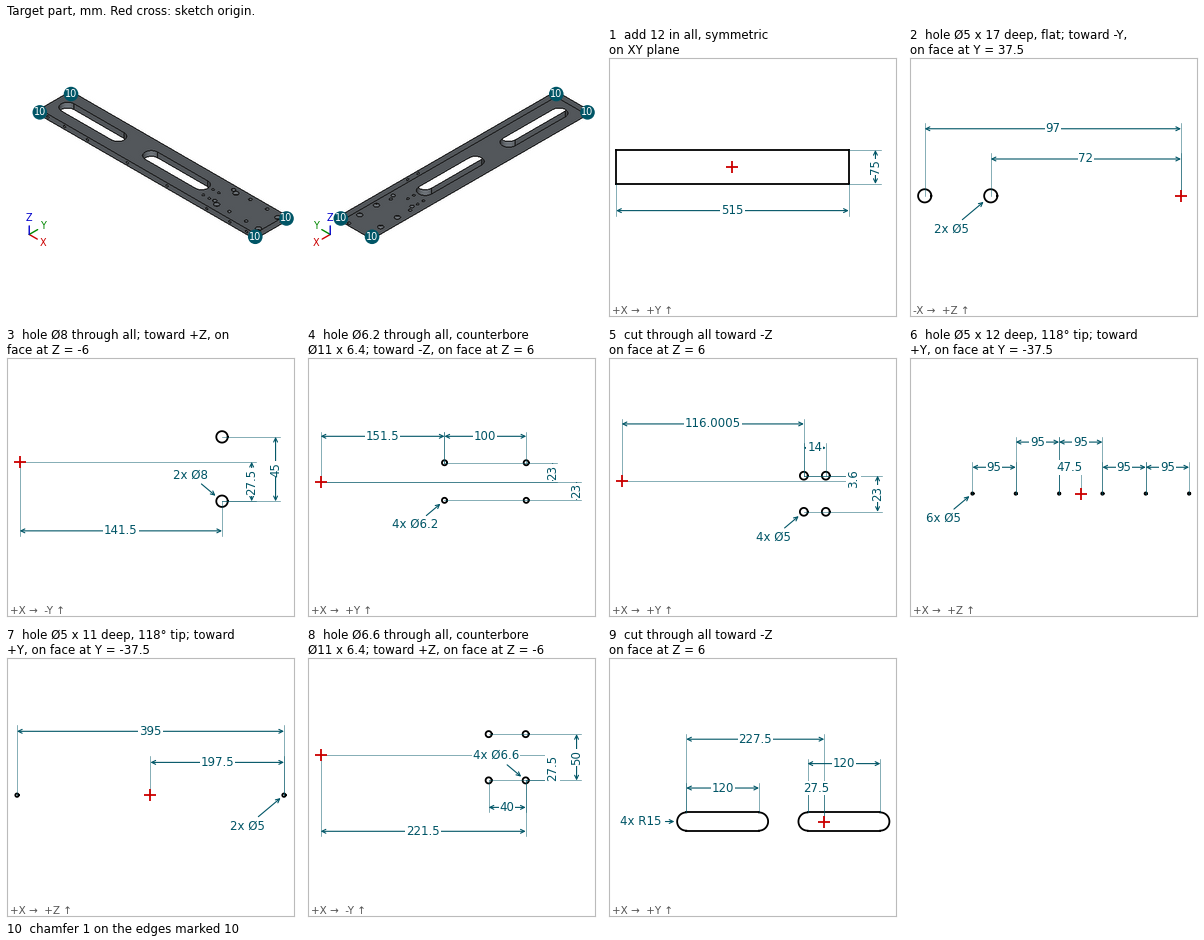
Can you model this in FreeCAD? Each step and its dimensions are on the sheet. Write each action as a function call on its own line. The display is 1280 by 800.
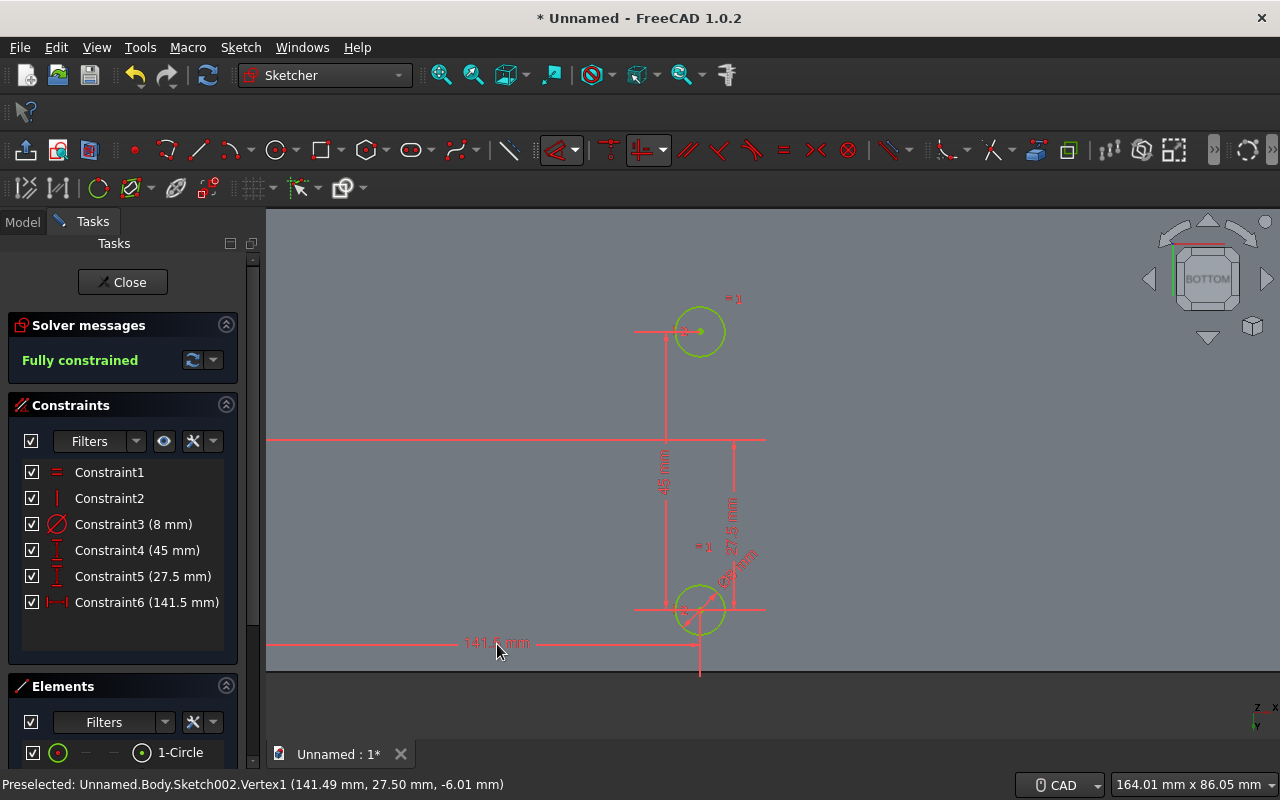
click(123, 282)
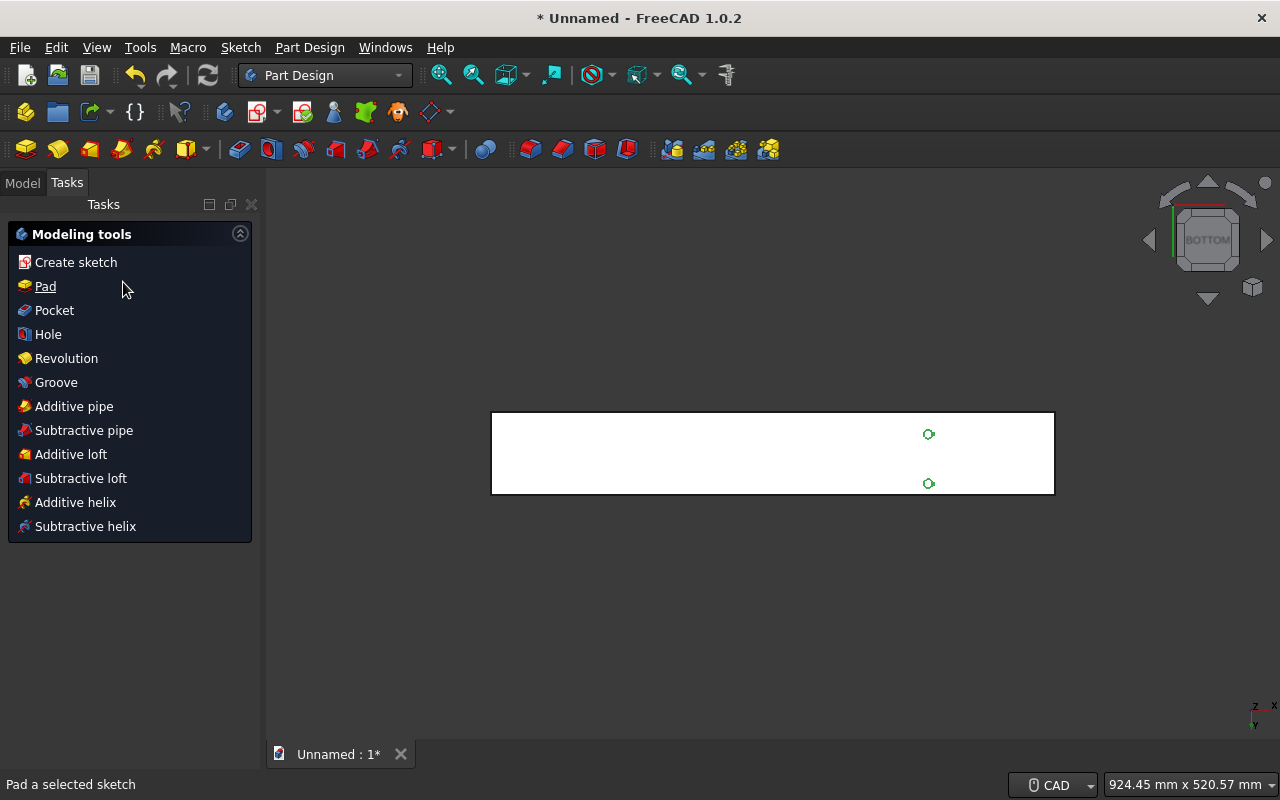
click(272, 150)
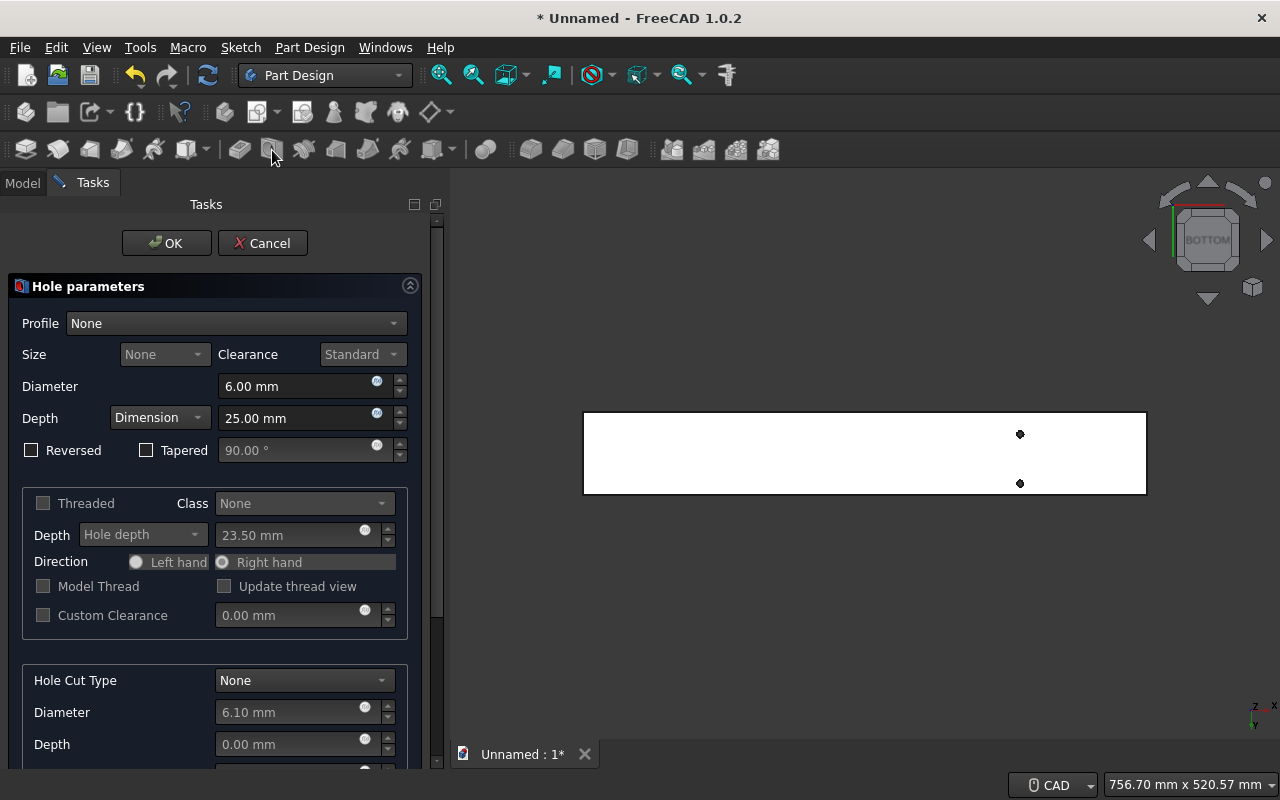
triple_click(305, 386)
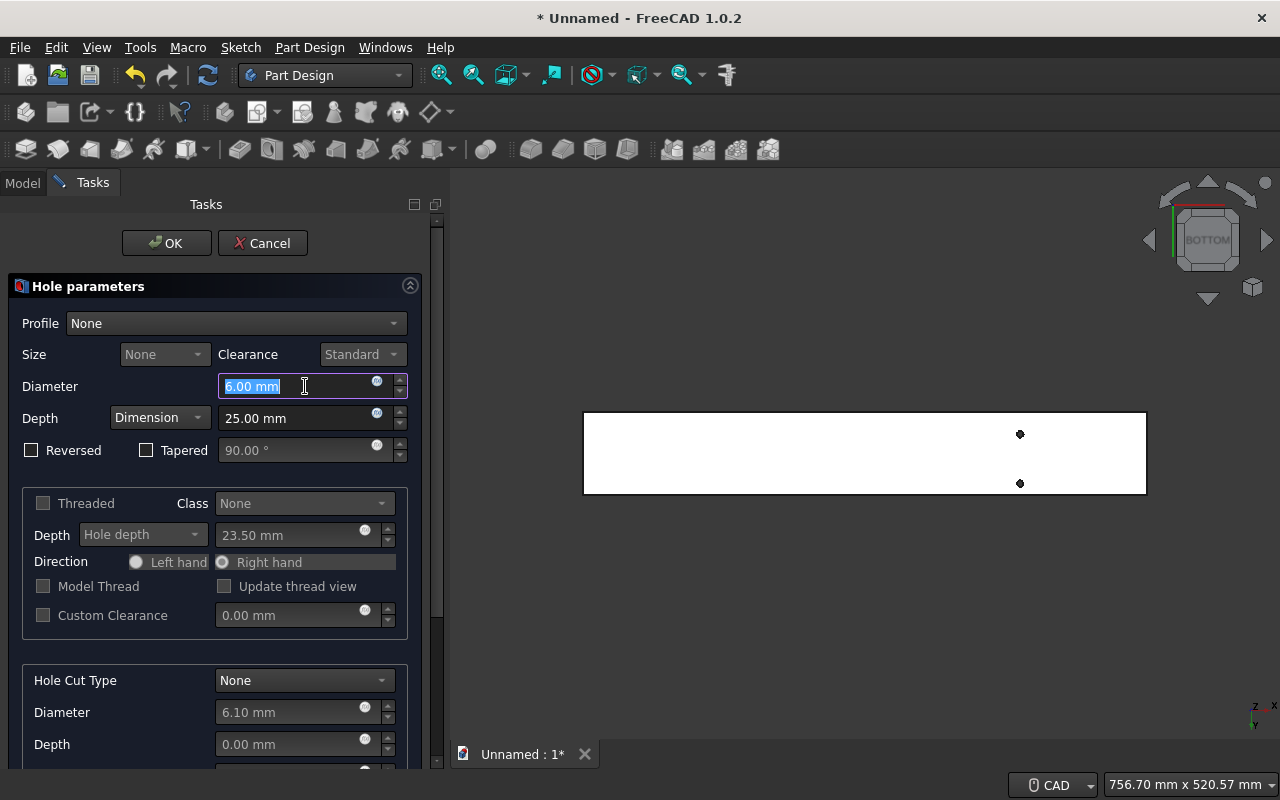
text(8)
key(Tab)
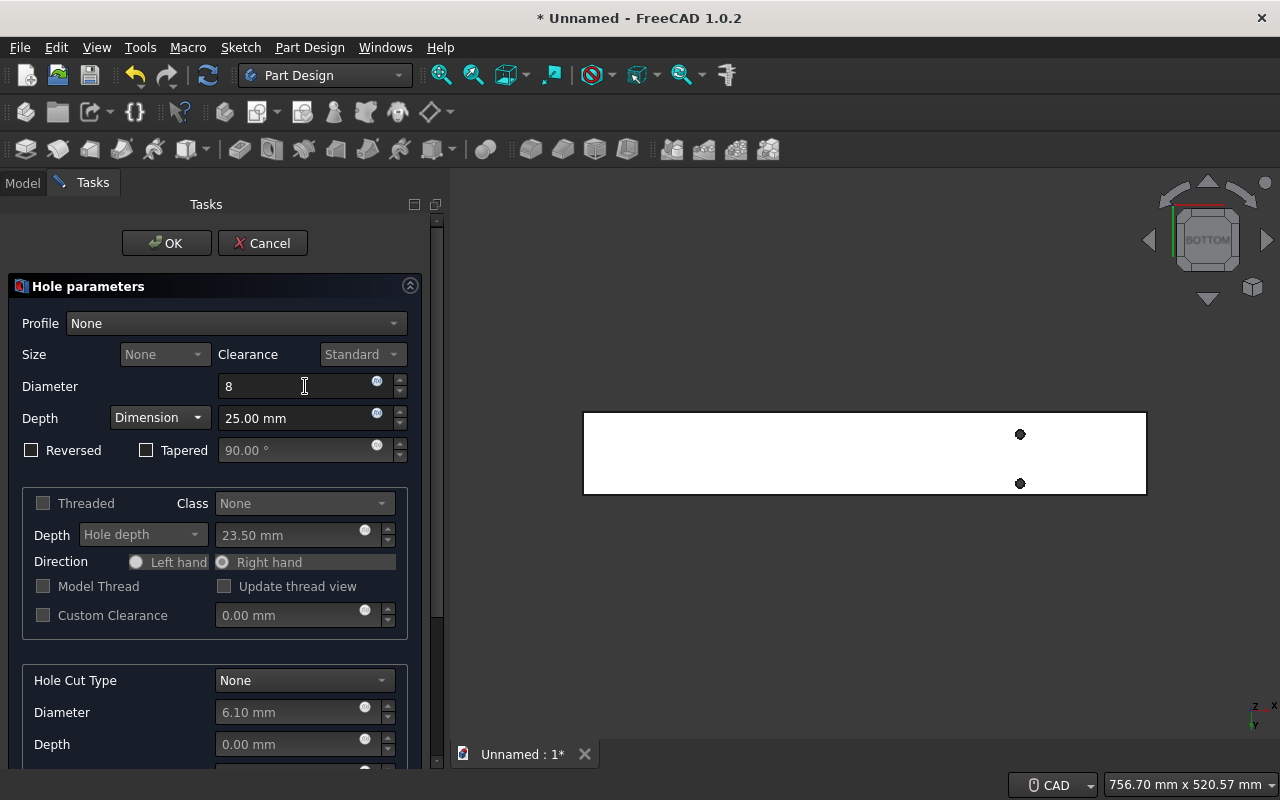
click(161, 418)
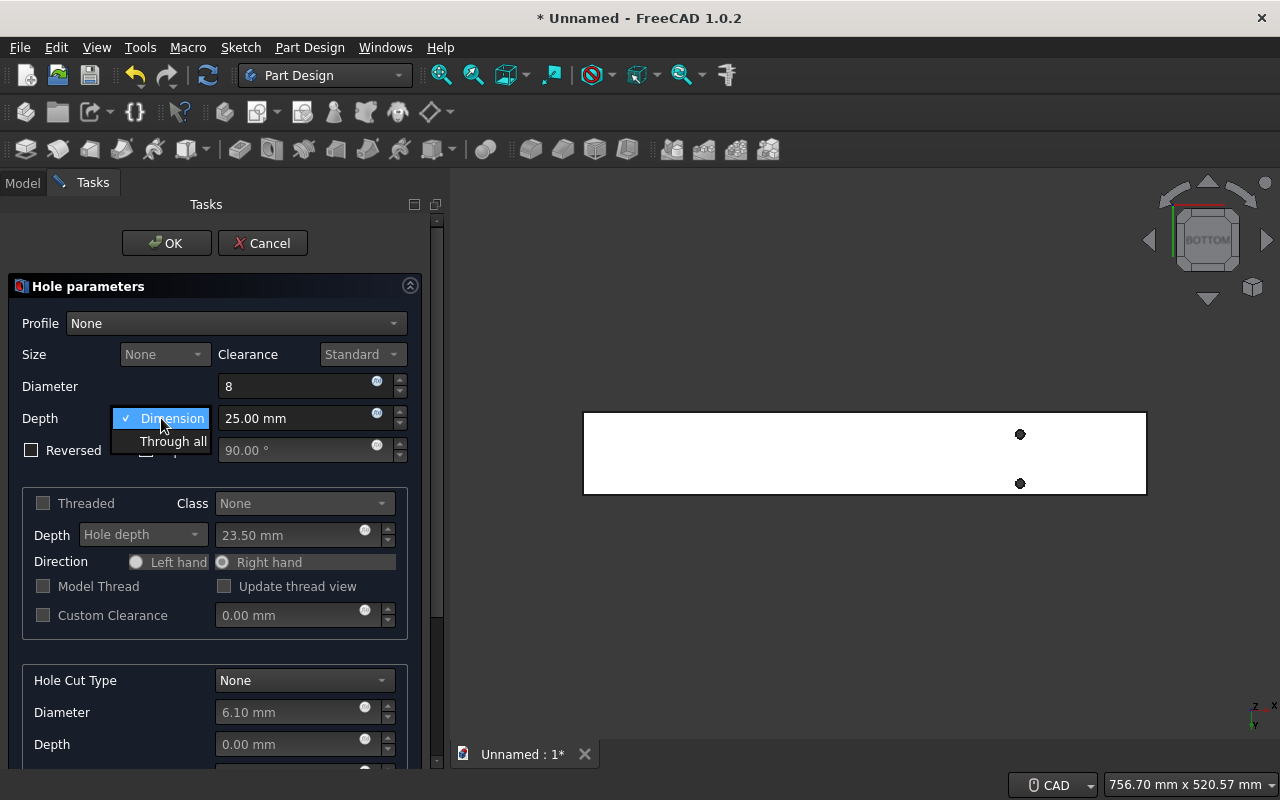
click(160, 442)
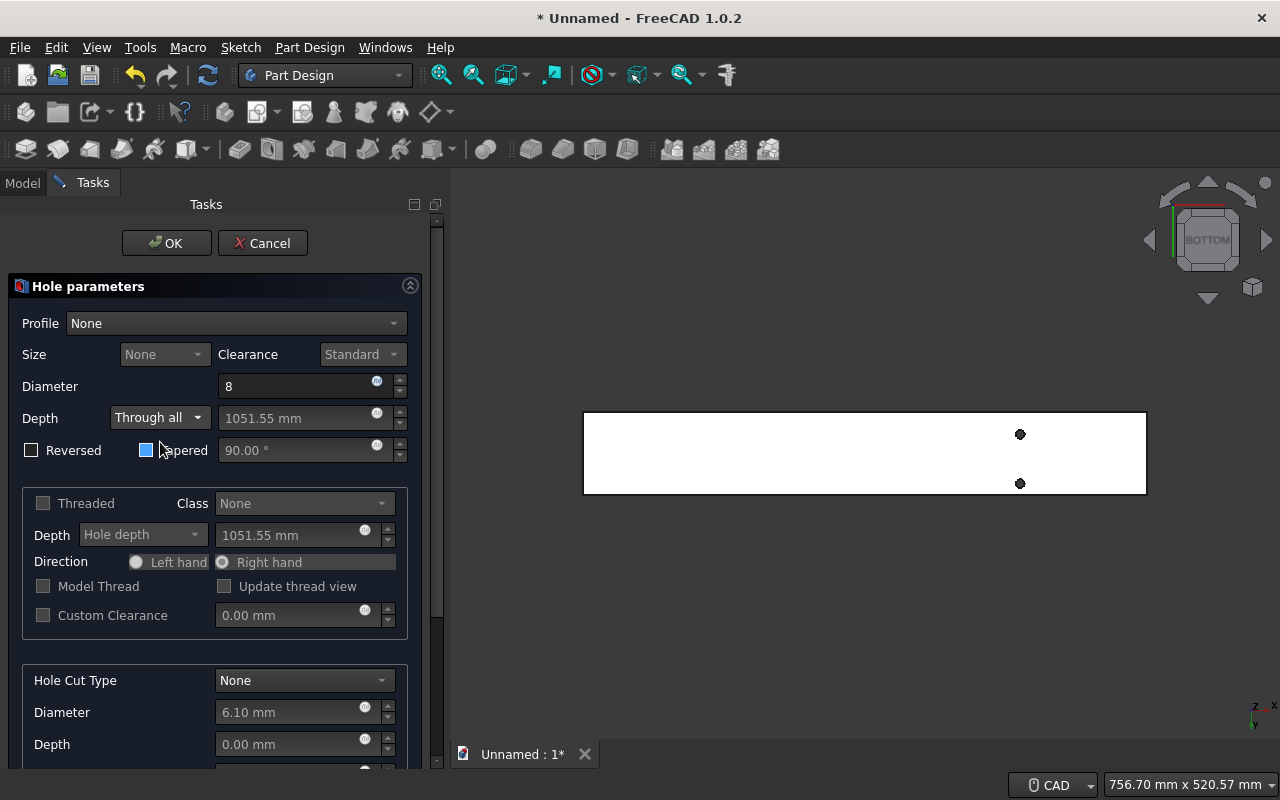
click(167, 243)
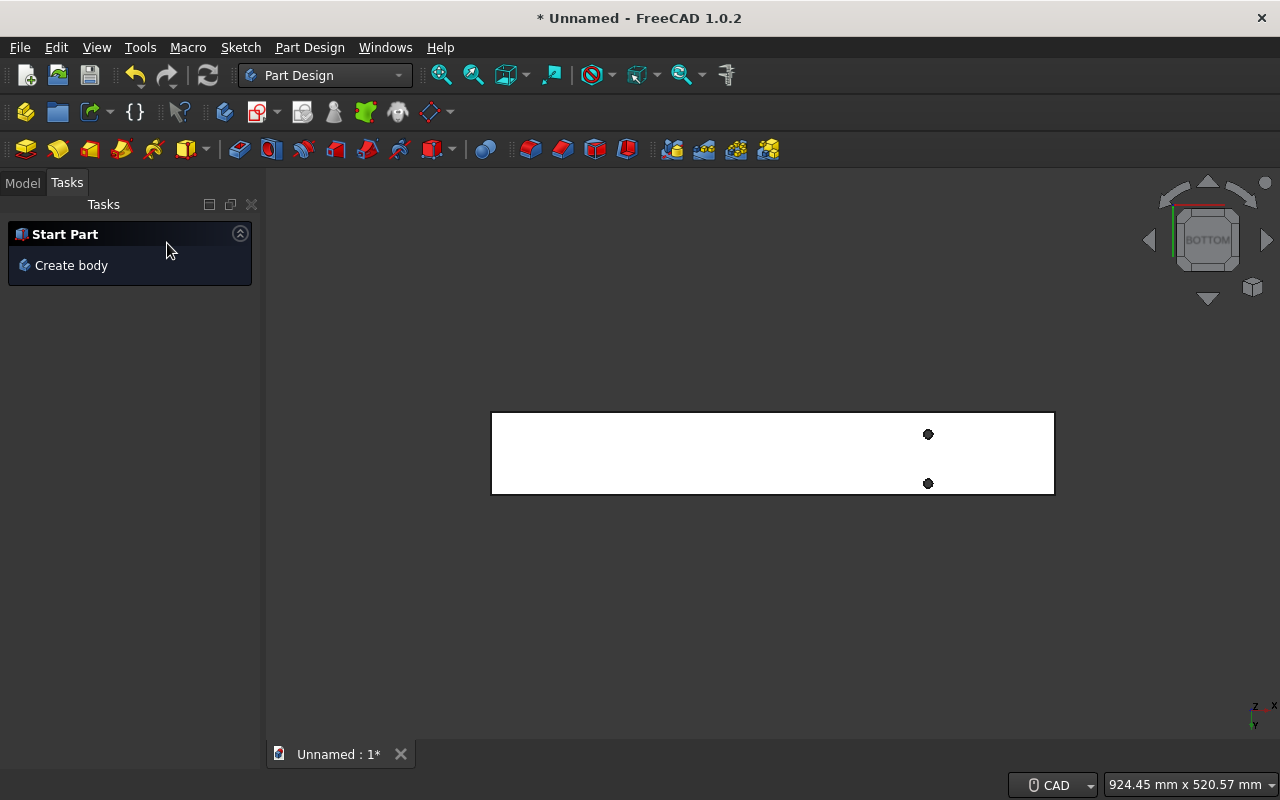
key(0)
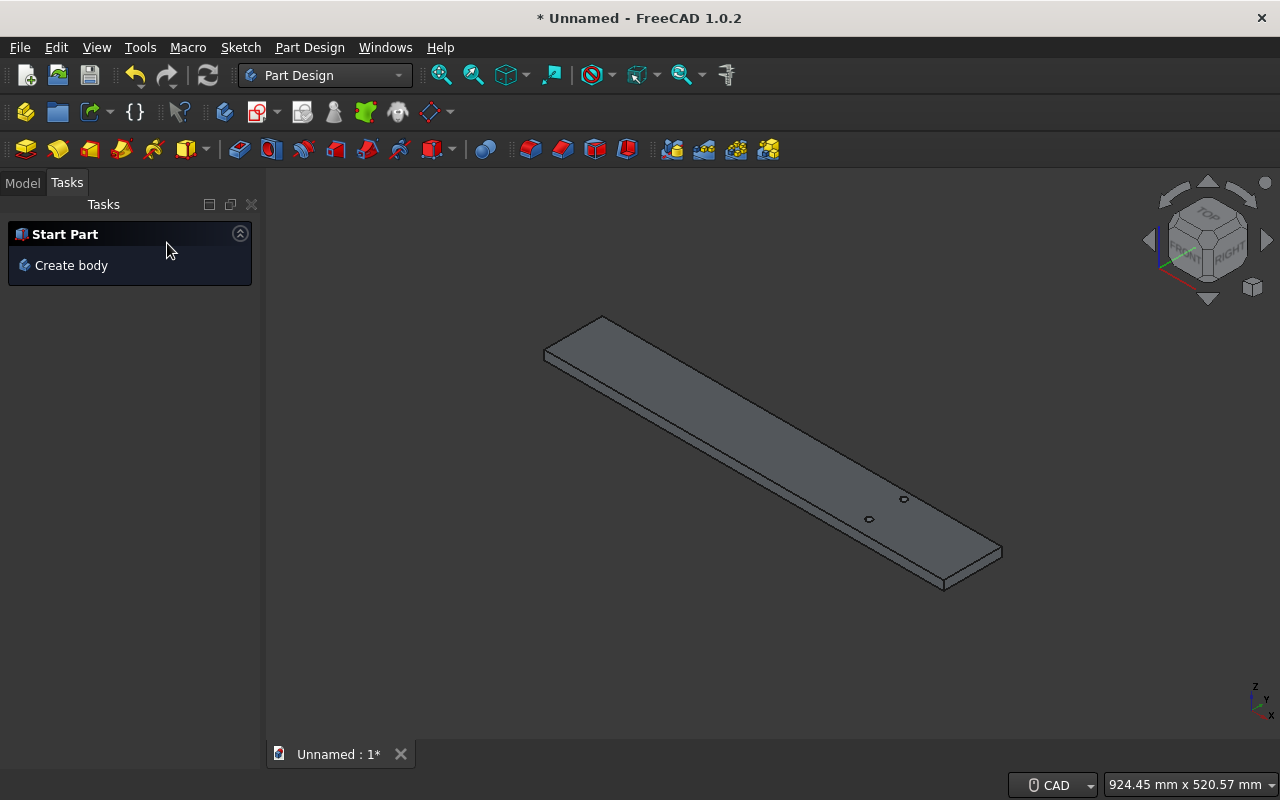
click(830, 480)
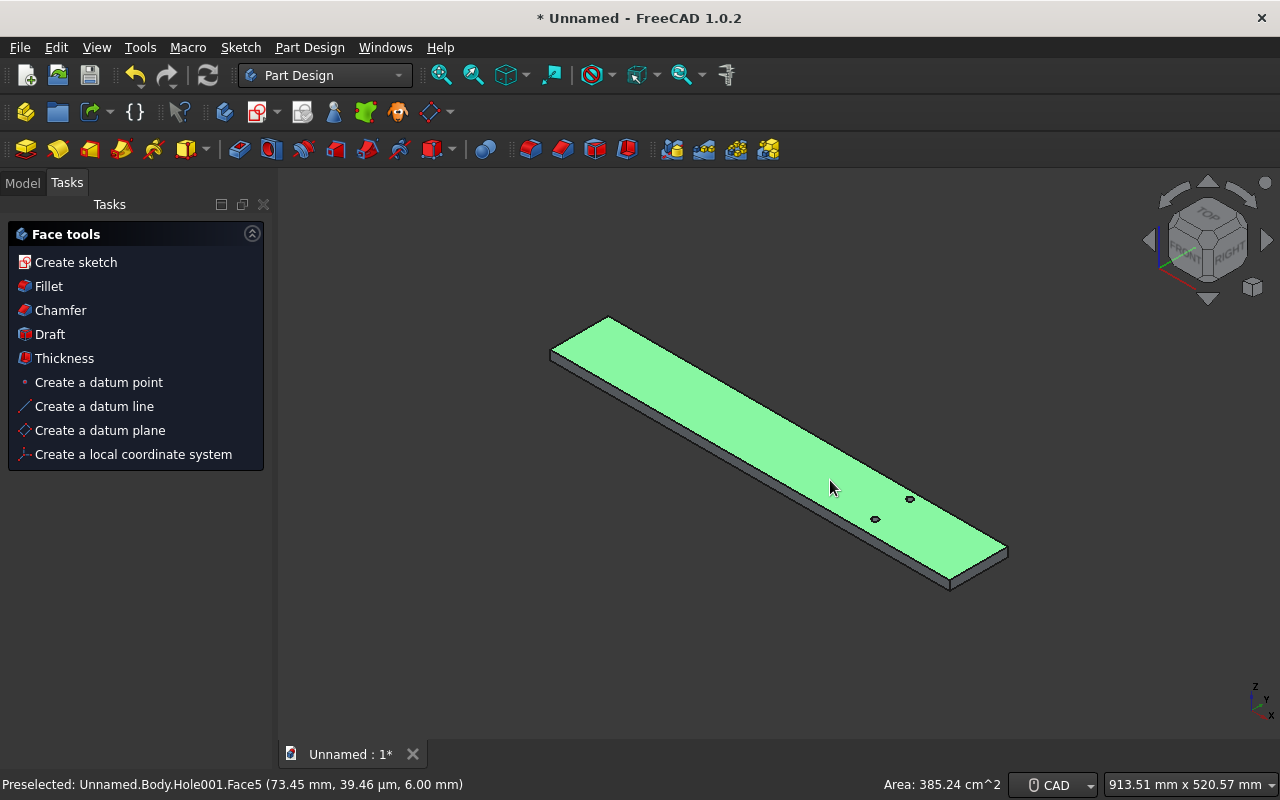
click(258, 112)